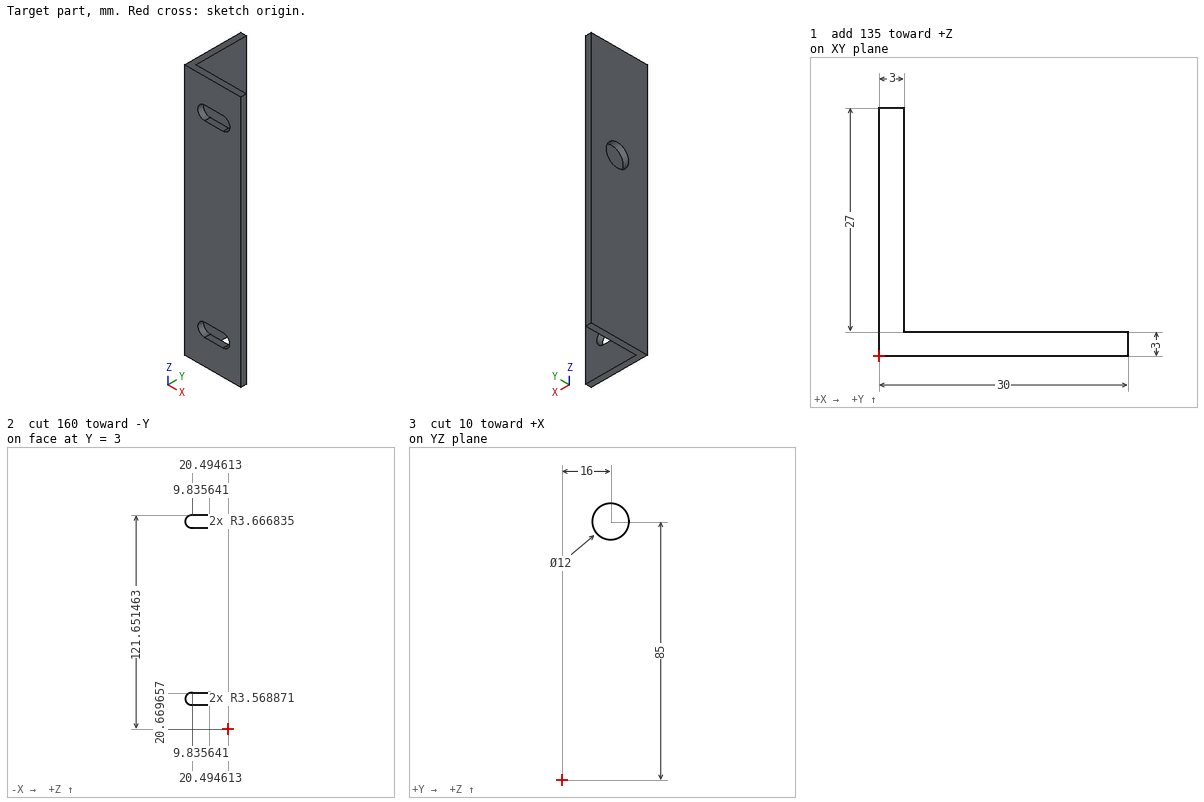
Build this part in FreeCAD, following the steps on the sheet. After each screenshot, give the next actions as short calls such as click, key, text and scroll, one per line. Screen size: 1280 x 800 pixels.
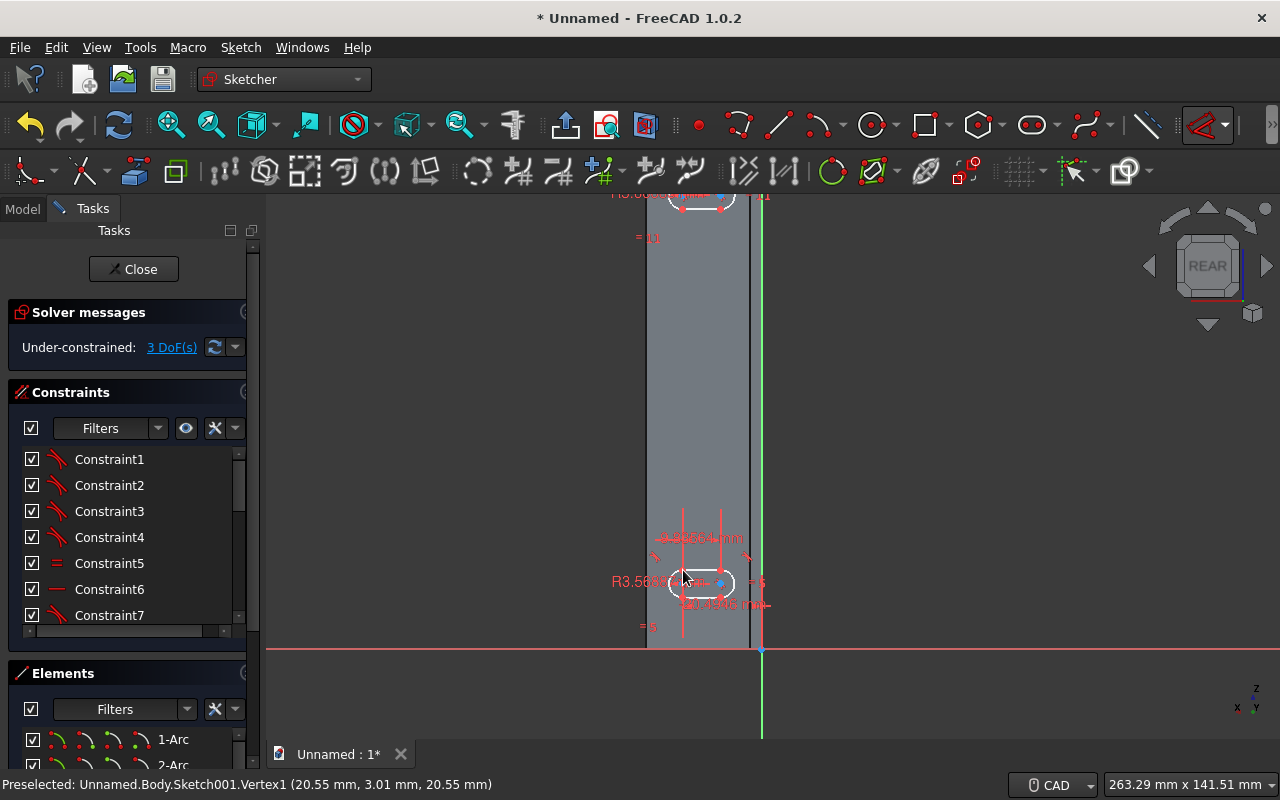
click(683, 570)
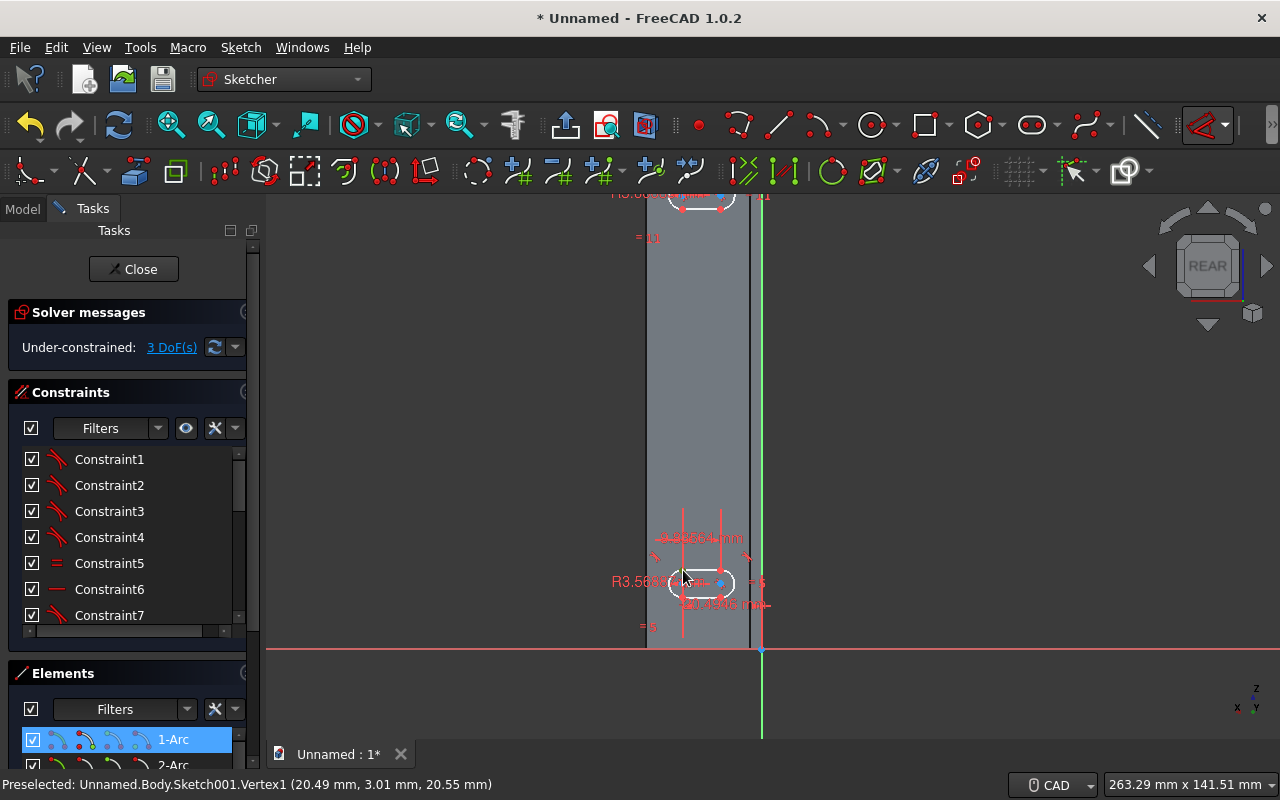
key(i)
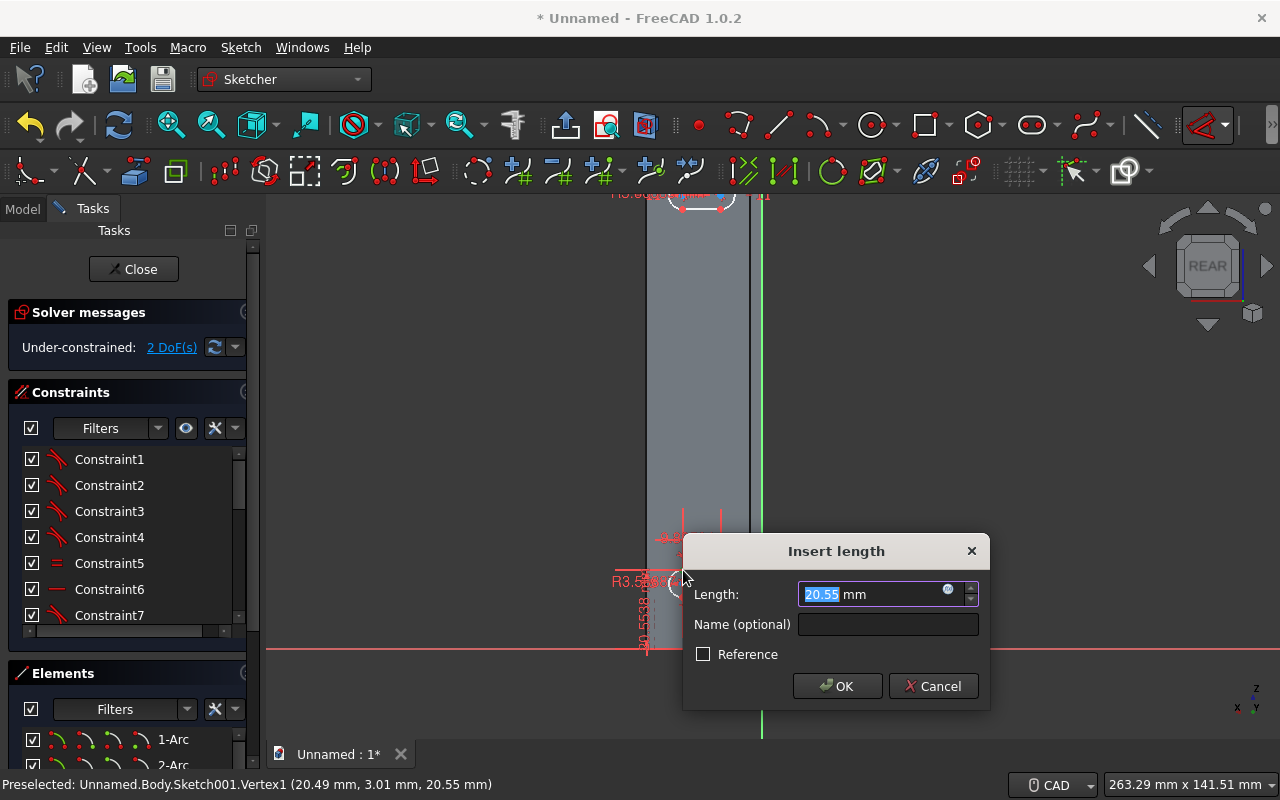
text(20.669657)
key(Return)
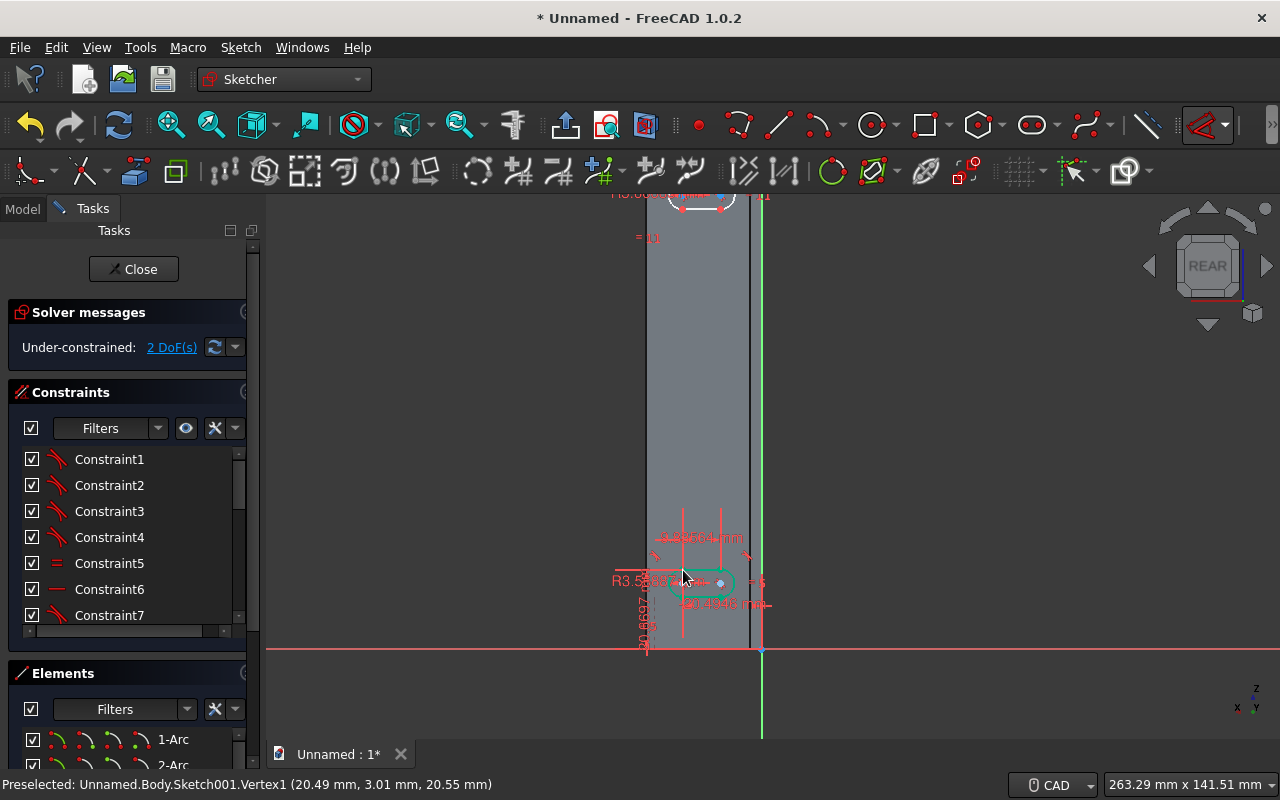
scroll(683, 571, down, 2)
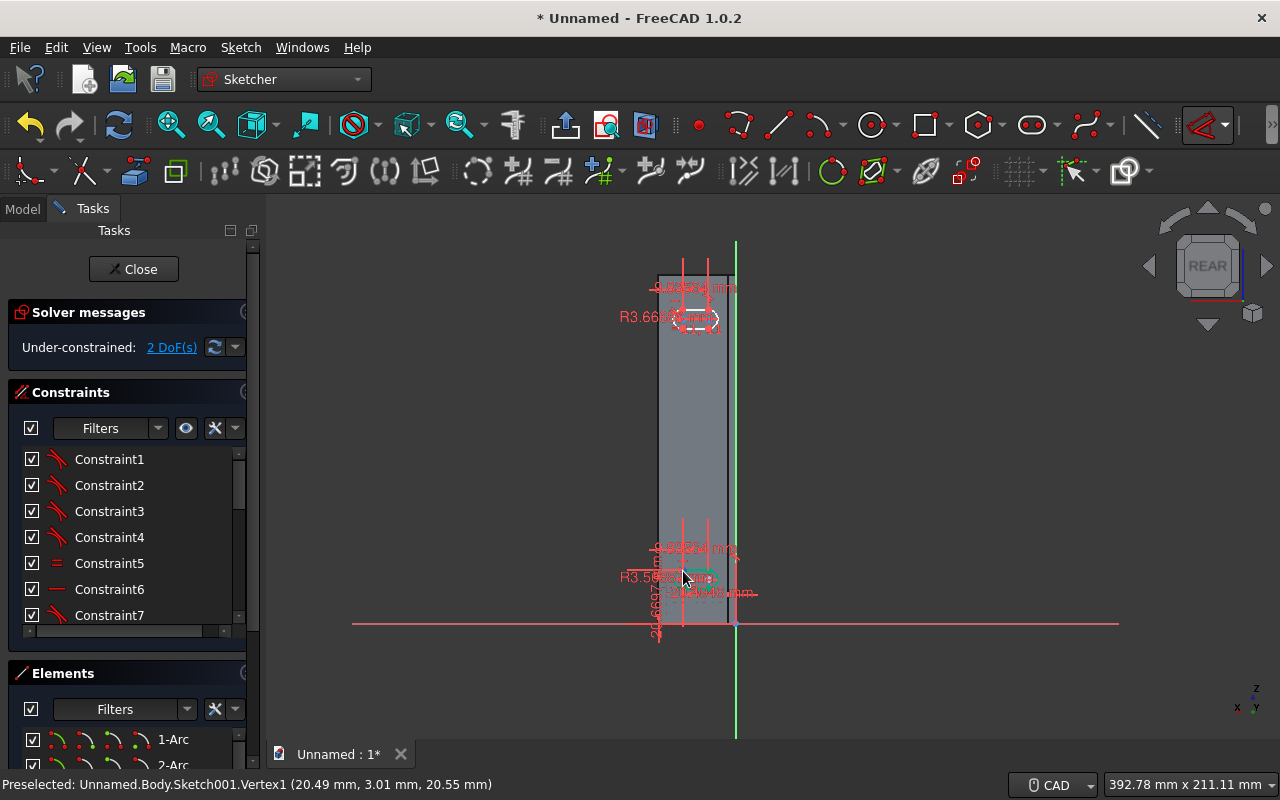
scroll(683, 310, up, 2)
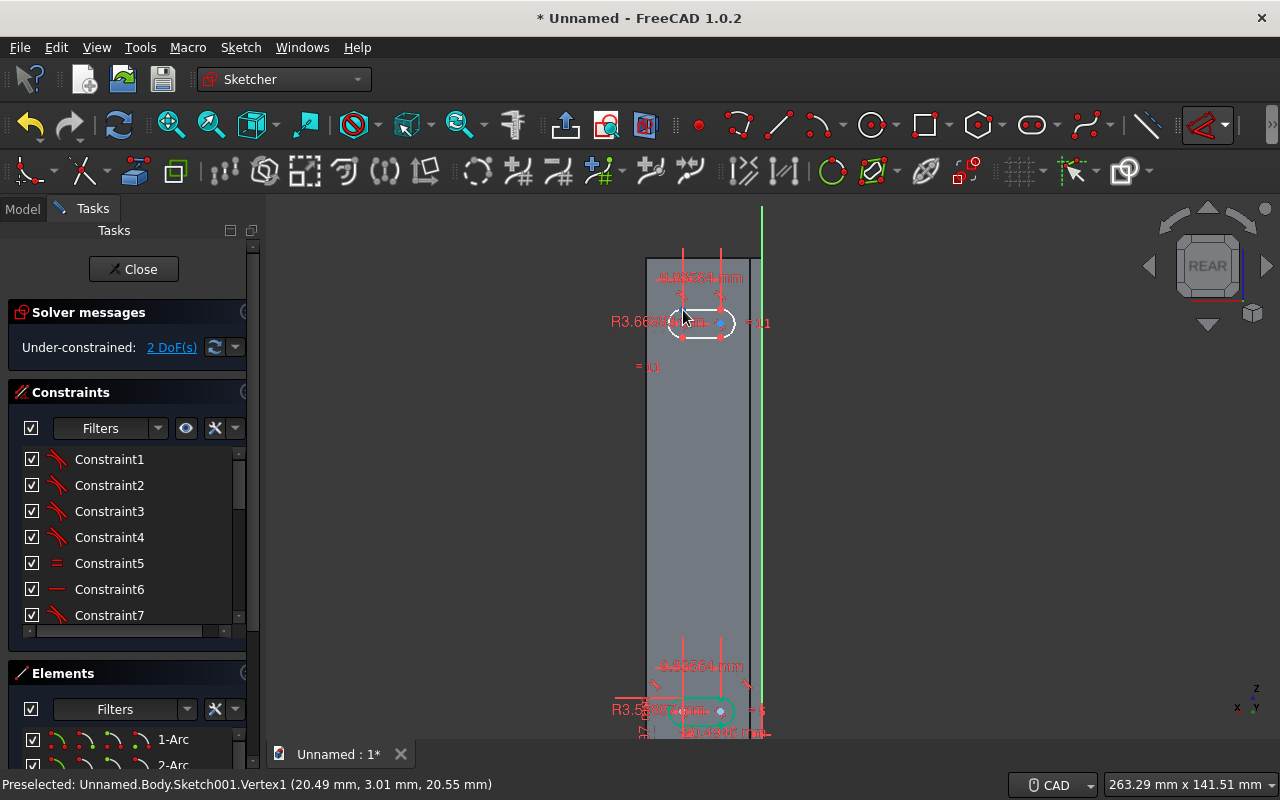
click(683, 310)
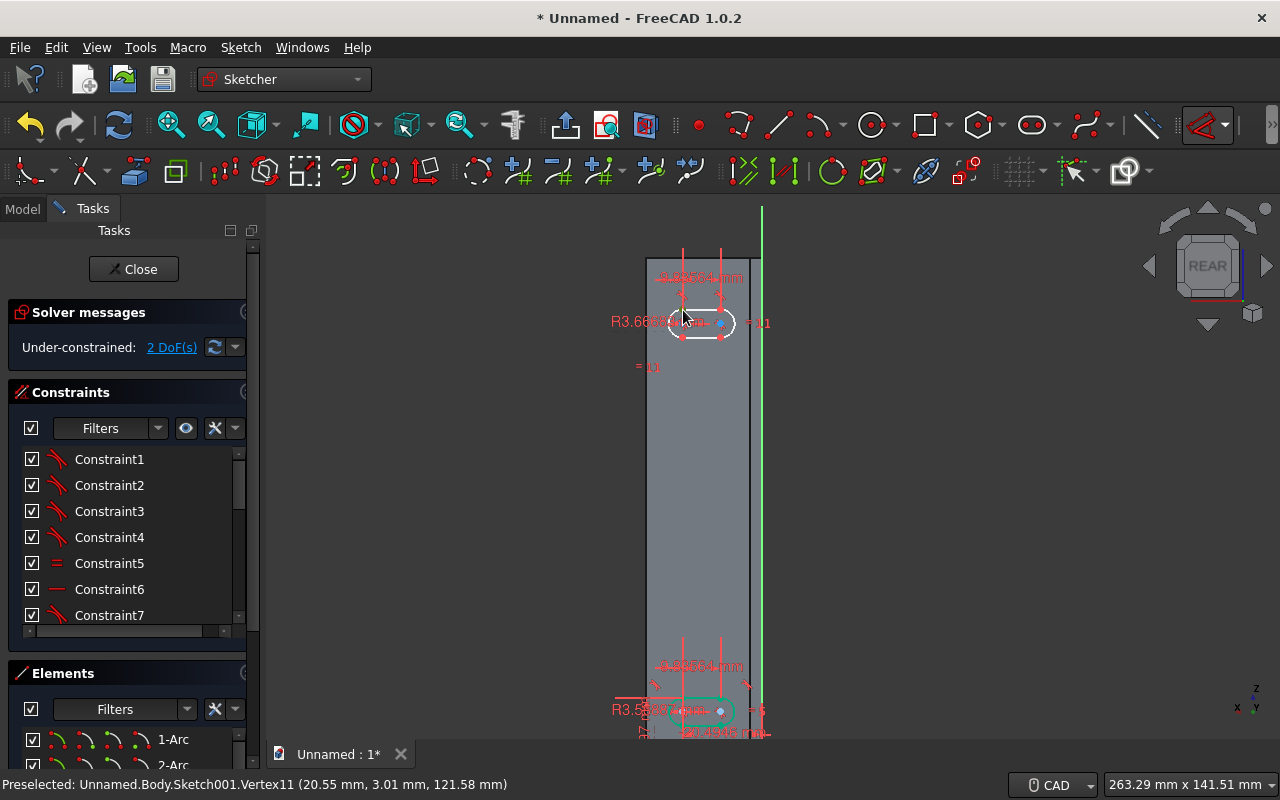
key(l)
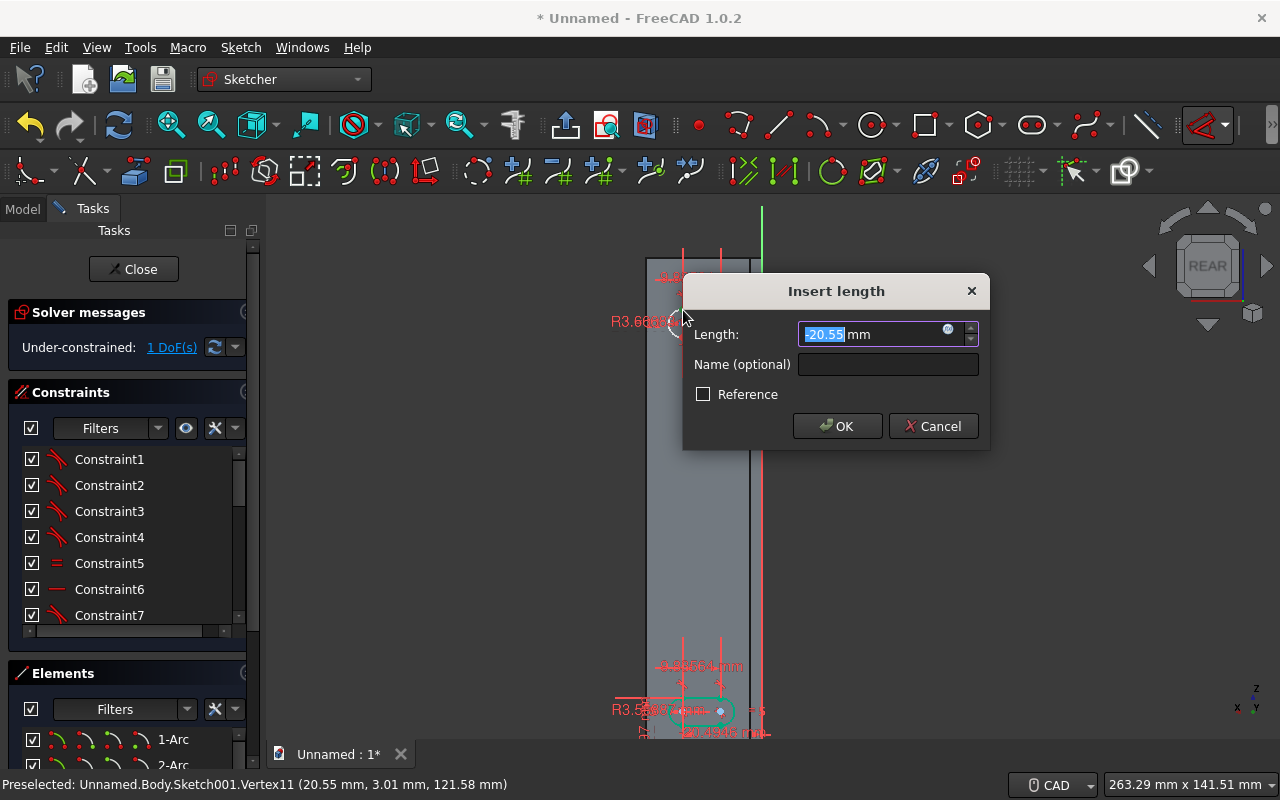
text(-20.494613)
key(Return)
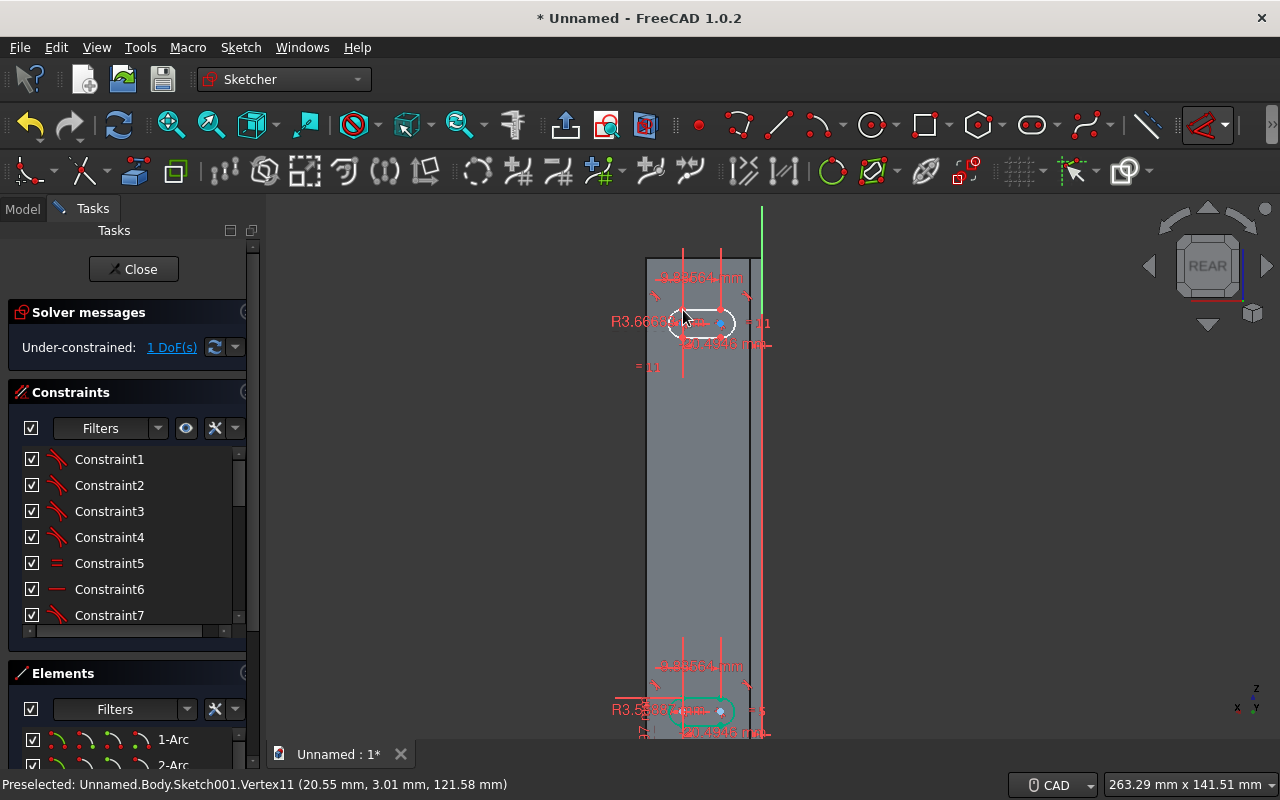
click(683, 310)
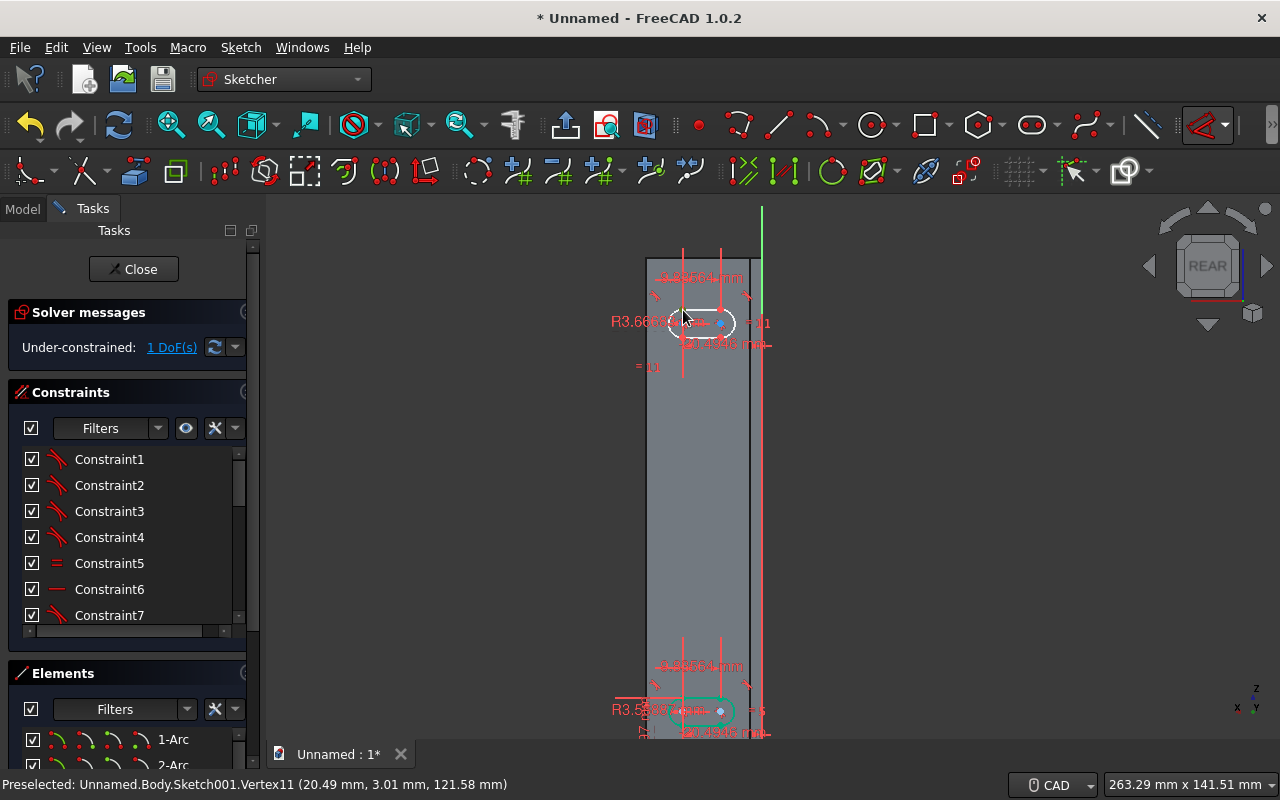
key(i)